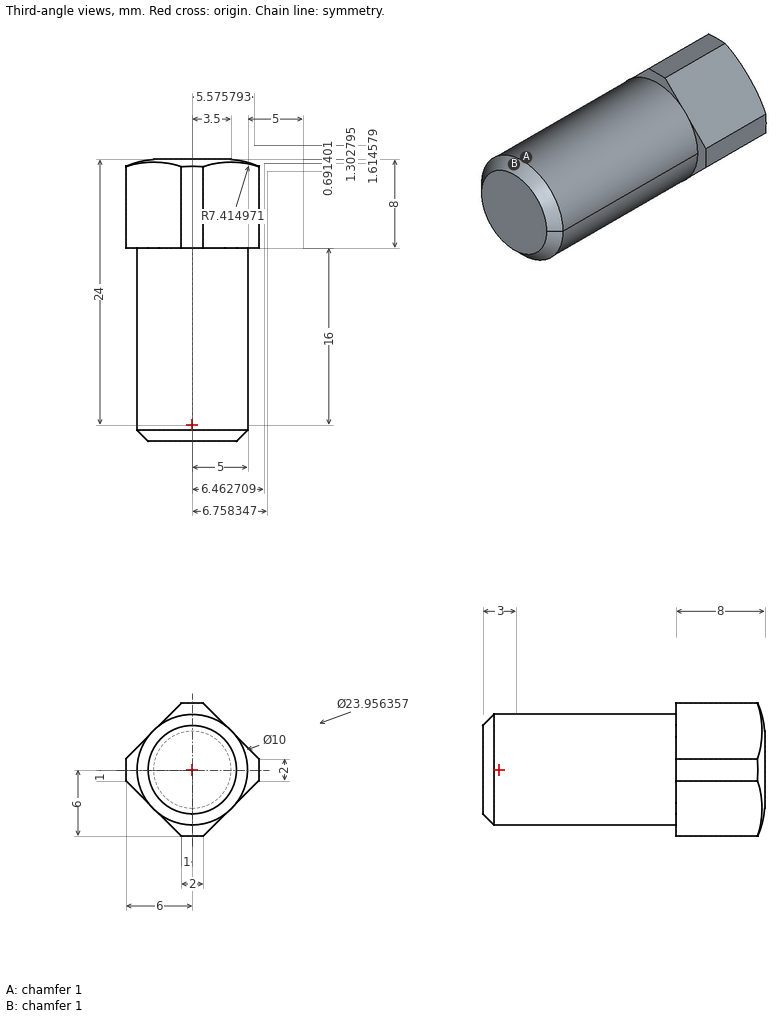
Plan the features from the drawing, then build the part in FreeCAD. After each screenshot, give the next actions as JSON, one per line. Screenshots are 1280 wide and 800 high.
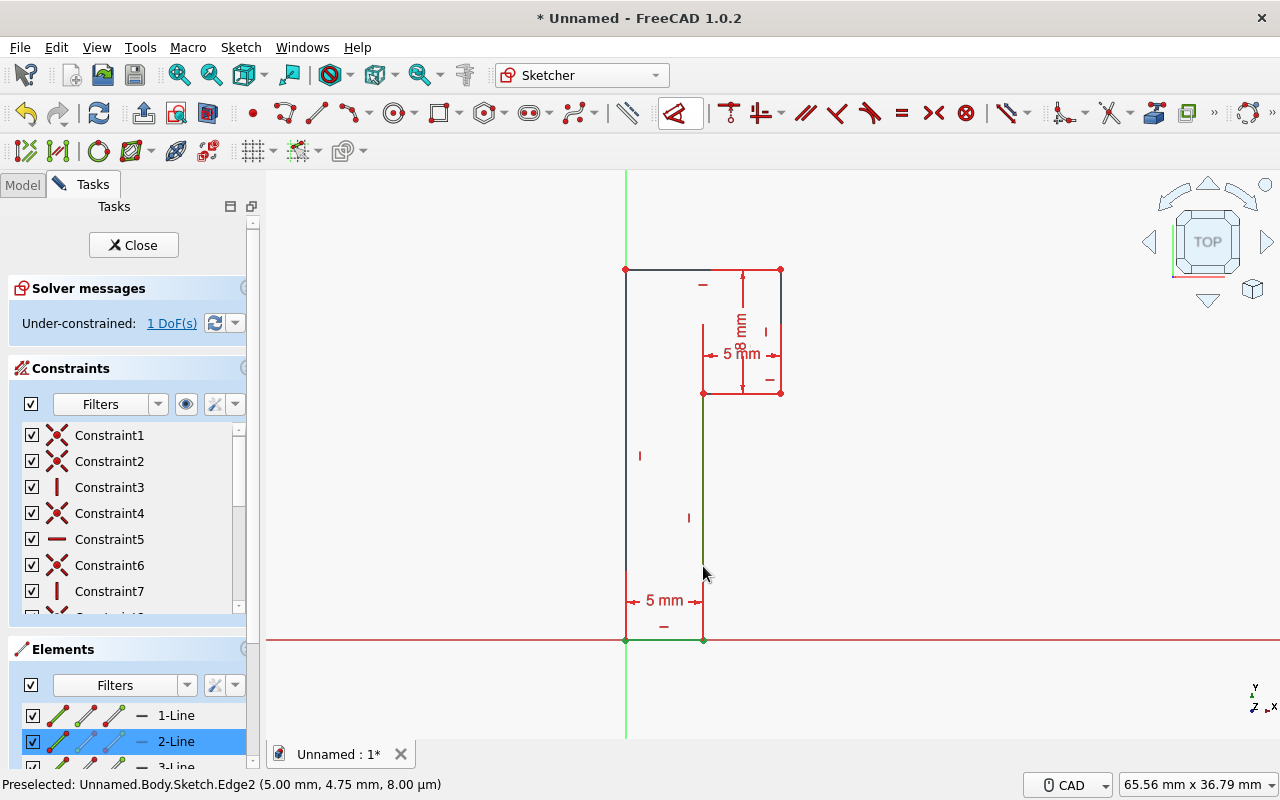
{"action": "key", "text": "i"}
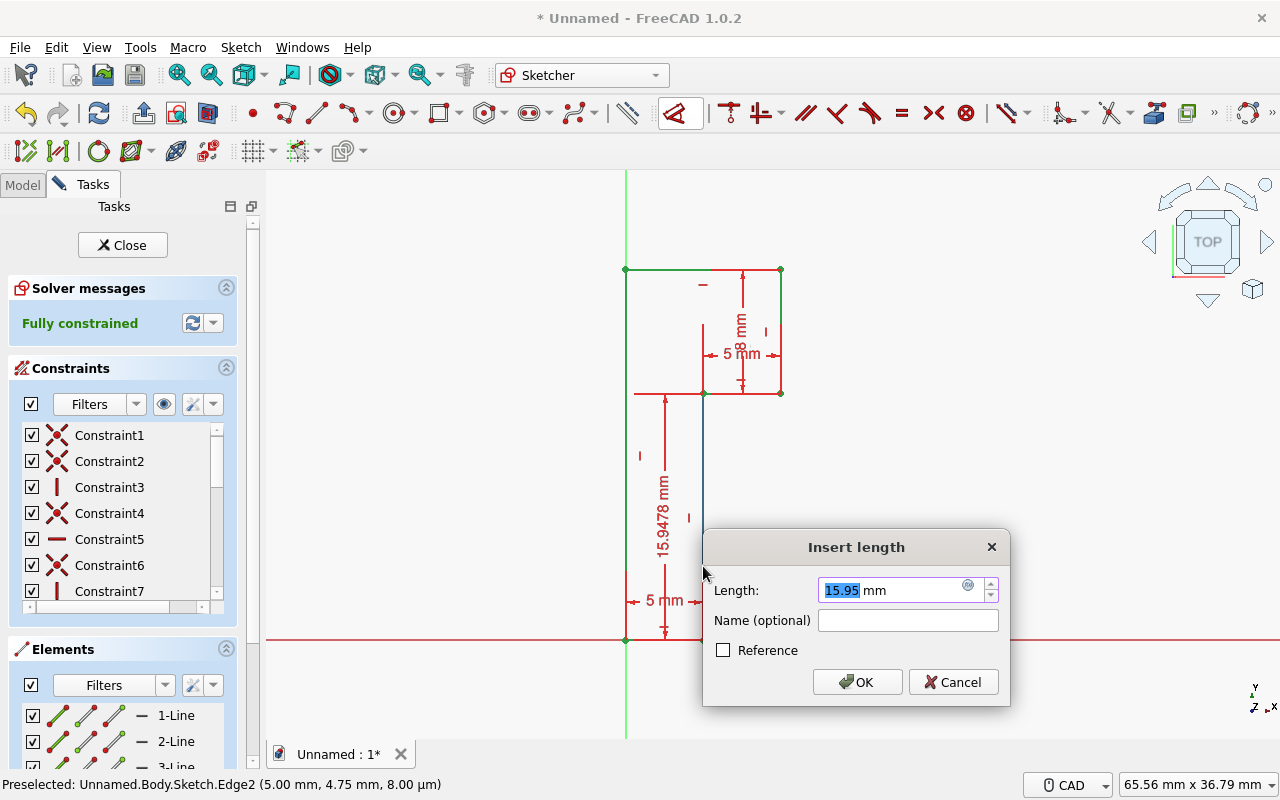
{"action": "type", "text": "16"}
{"action": "key", "text": "Return"}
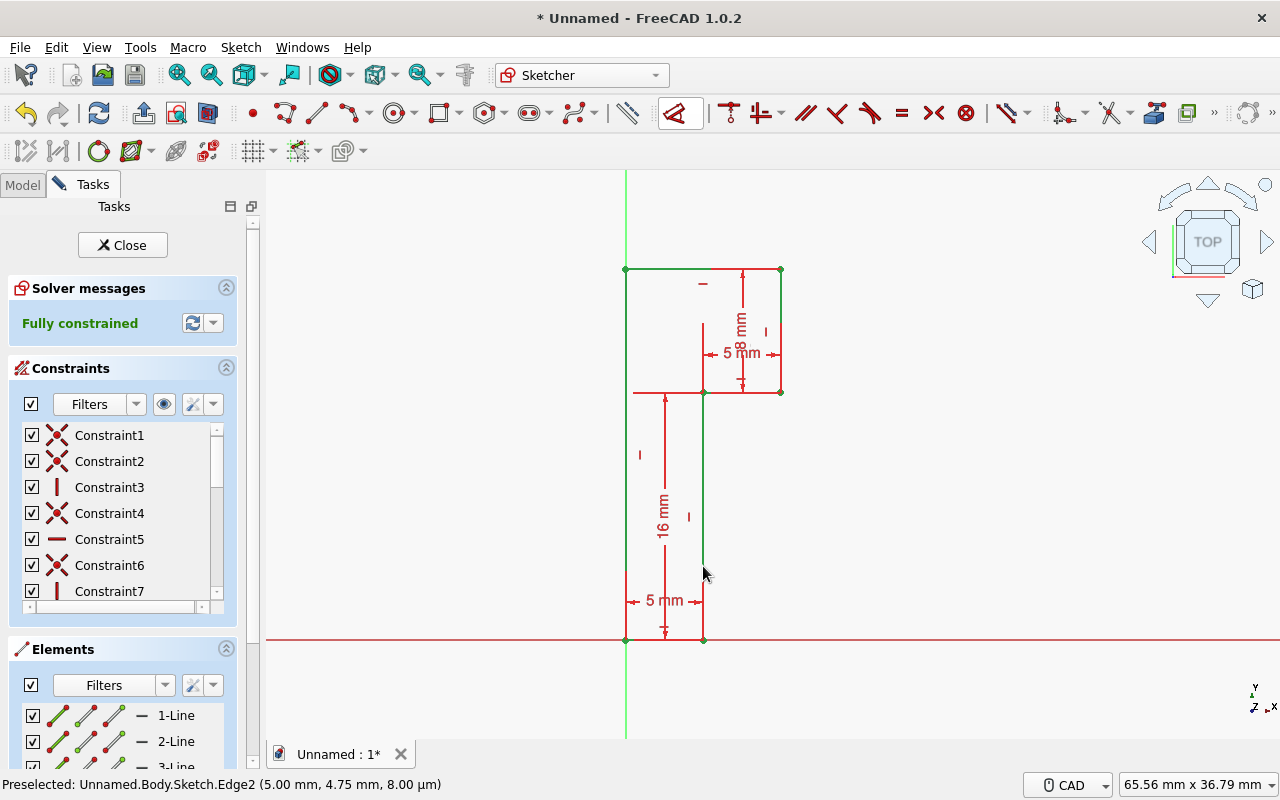
{"action": "left_click", "coordinate": [123, 245]}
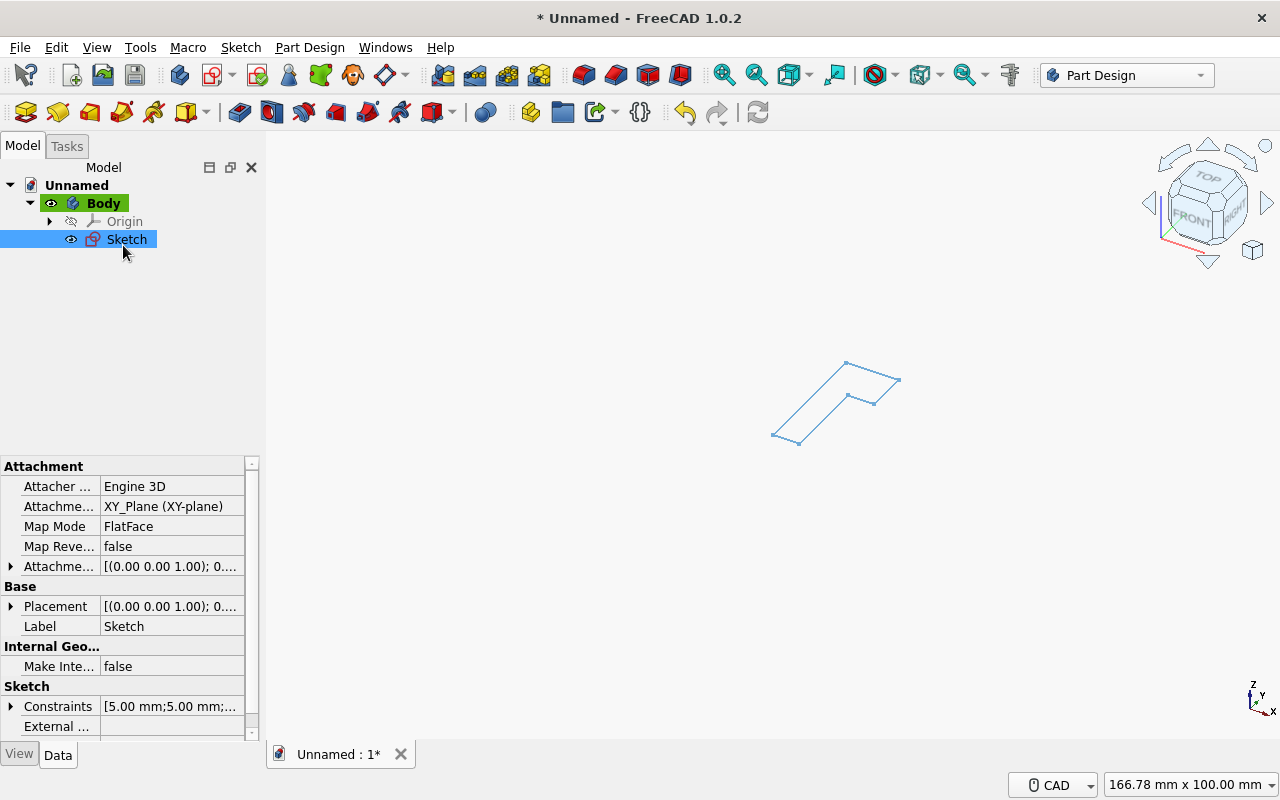
{"action": "left_click", "coordinate": [58, 112]}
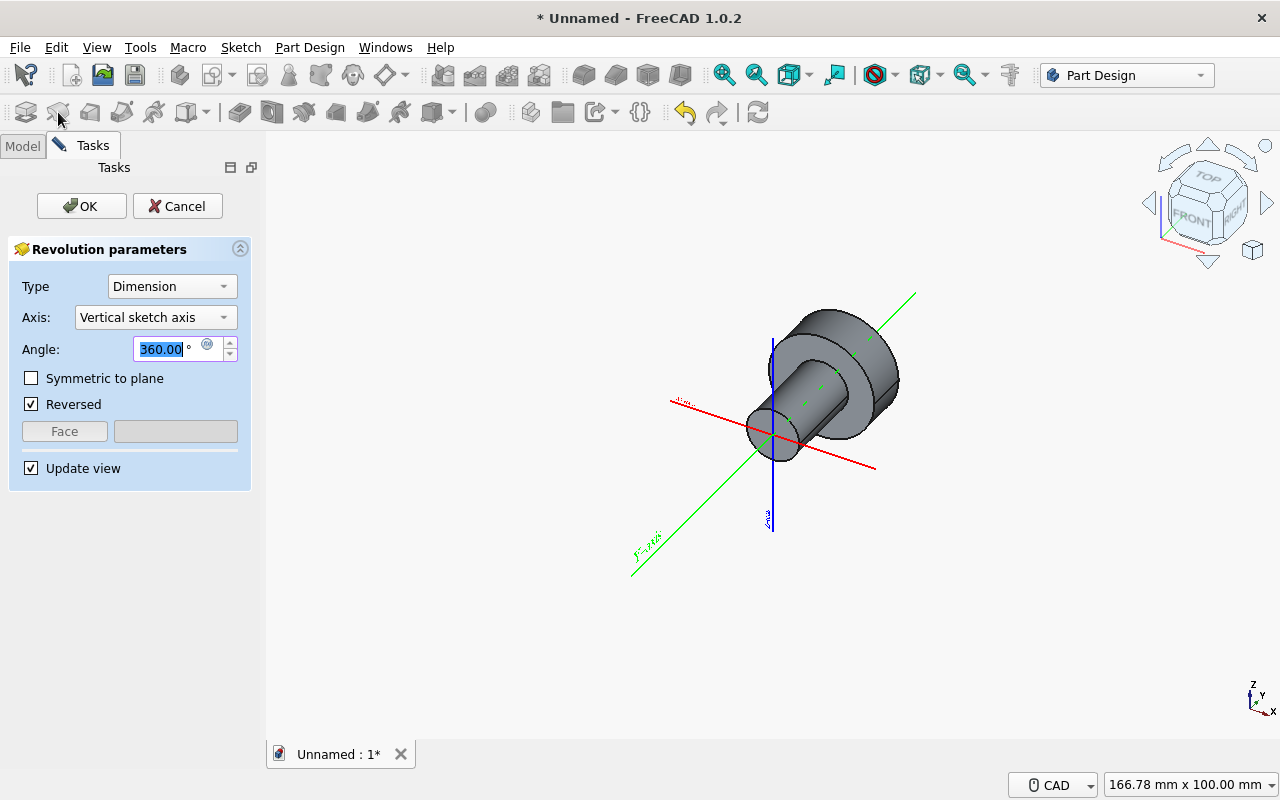
{"action": "left_click", "coordinate": [82, 206]}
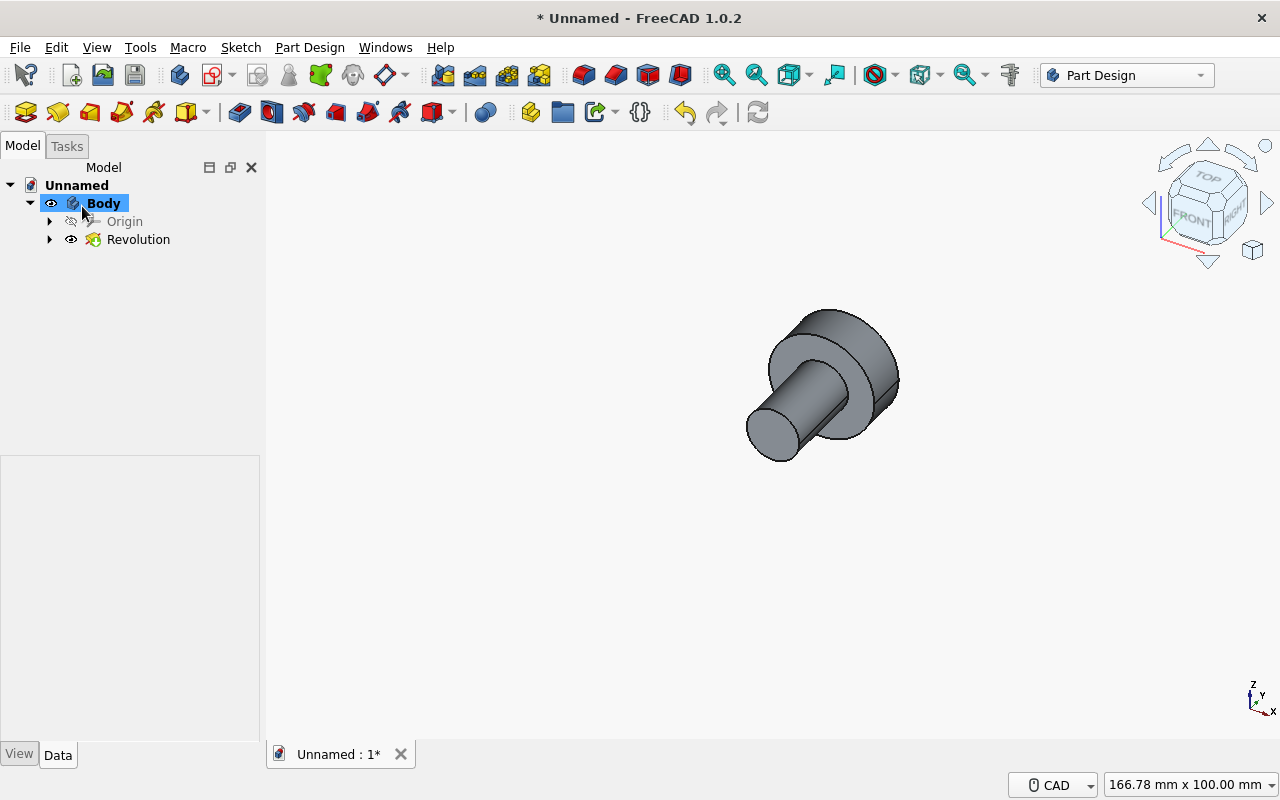
{"action": "left_click", "coordinate": [726, 76]}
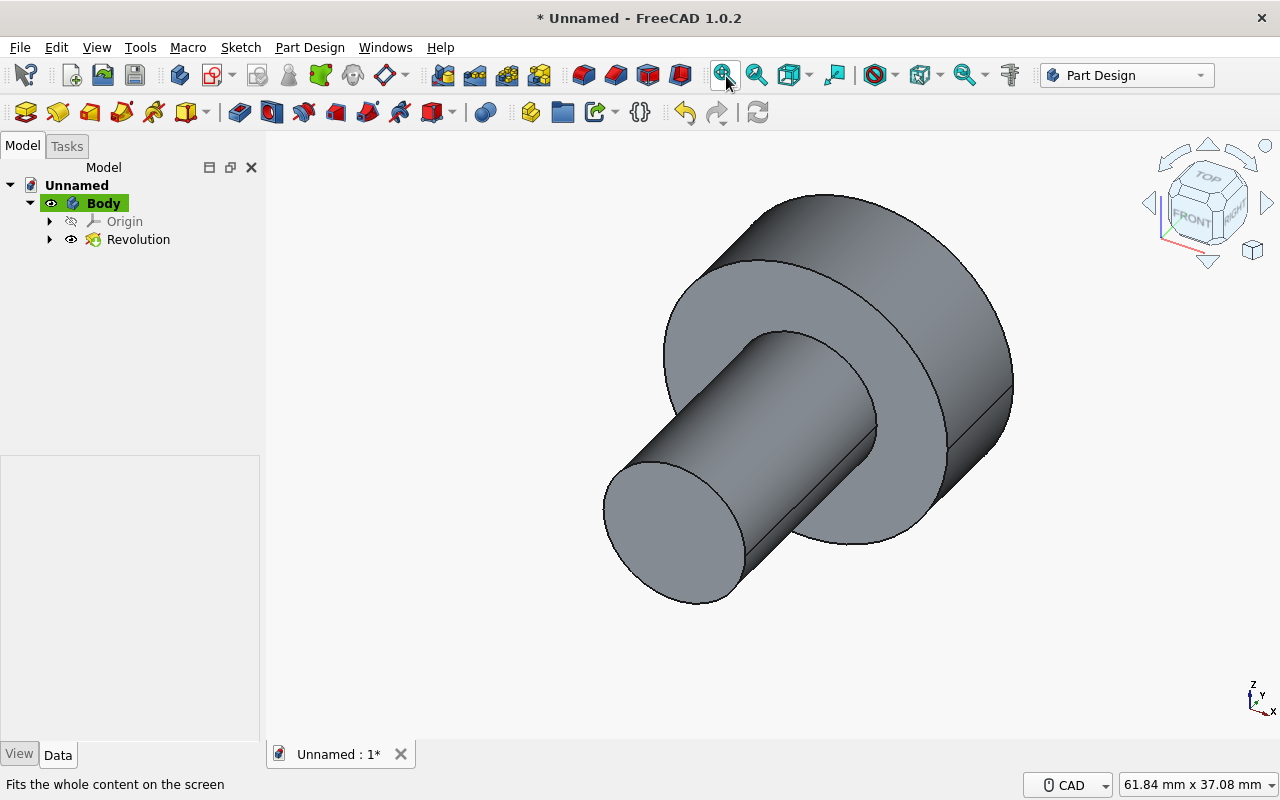
{"action": "left_click", "coordinate": [617, 473]}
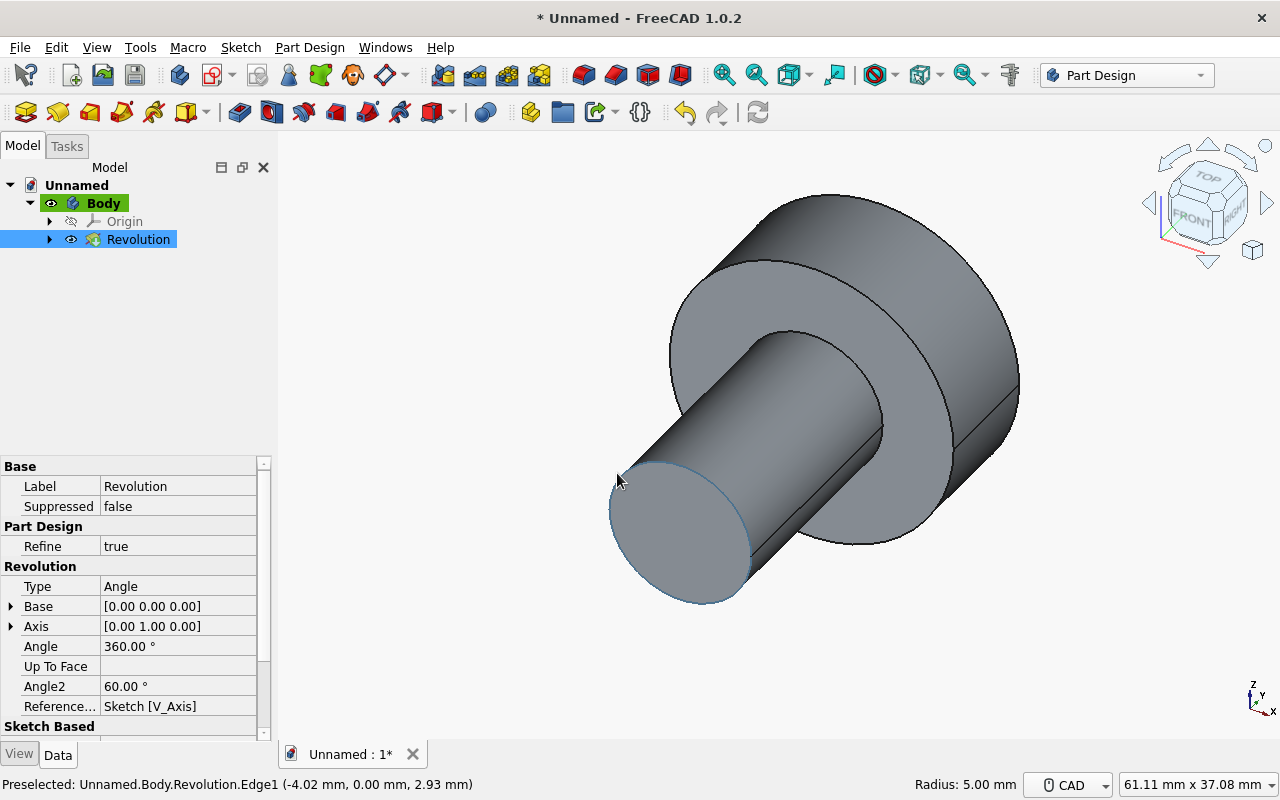
{"action": "left_click", "coordinate": [616, 76]}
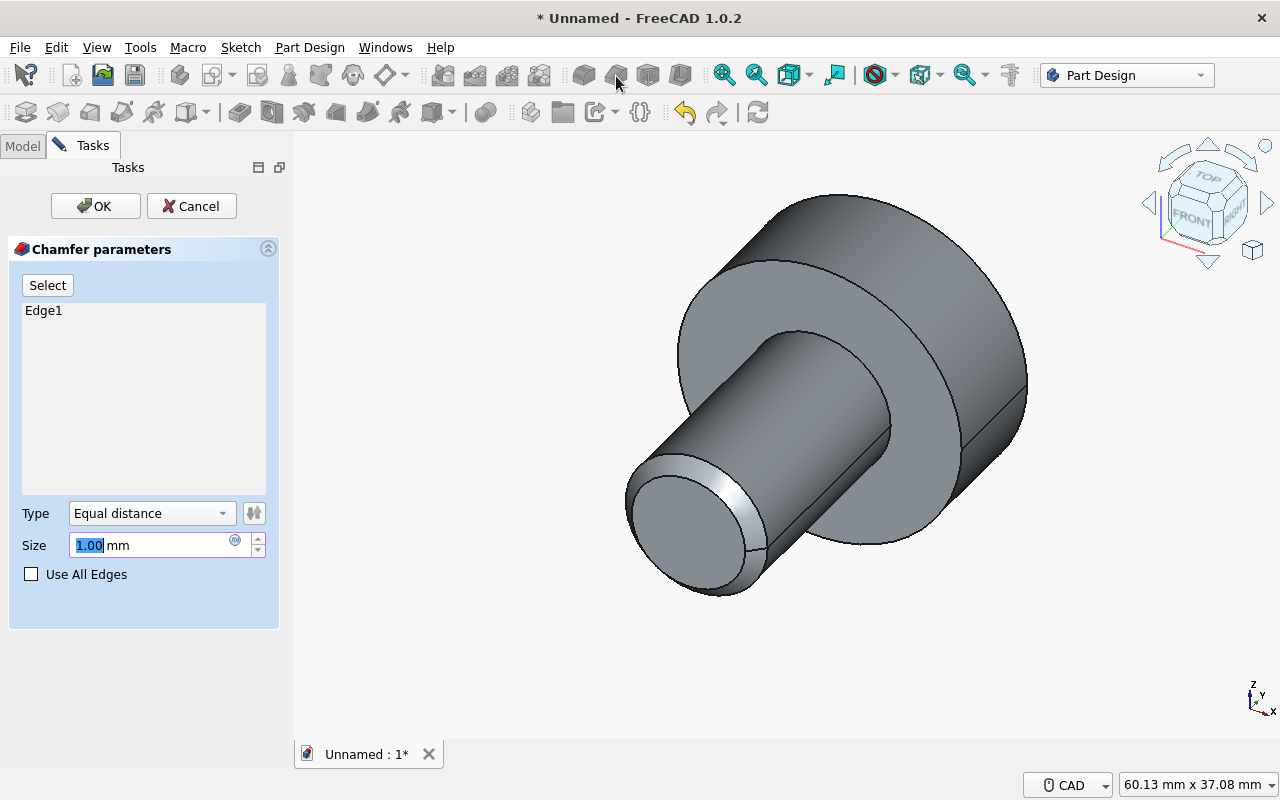
{"action": "type", "text": "1"}
{"action": "key", "text": "Tab"}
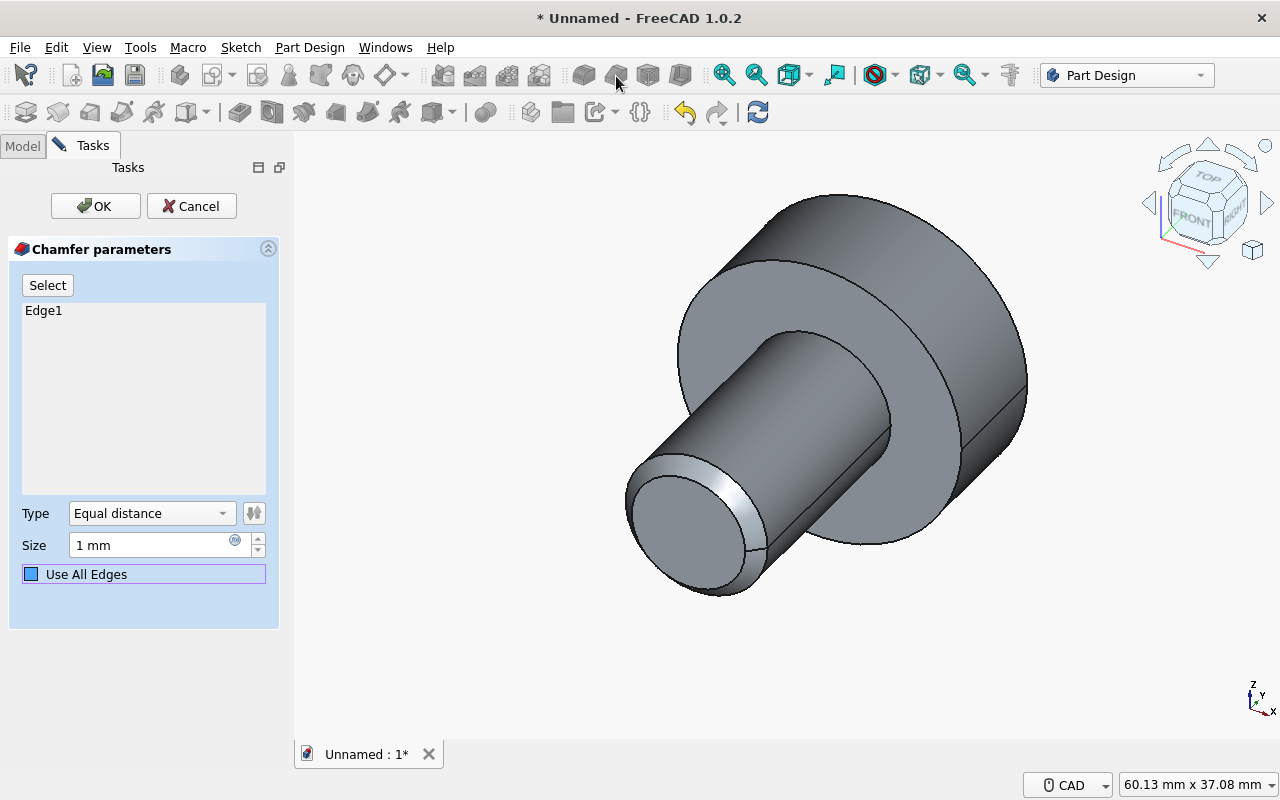
{"action": "left_click", "coordinate": [96, 206]}